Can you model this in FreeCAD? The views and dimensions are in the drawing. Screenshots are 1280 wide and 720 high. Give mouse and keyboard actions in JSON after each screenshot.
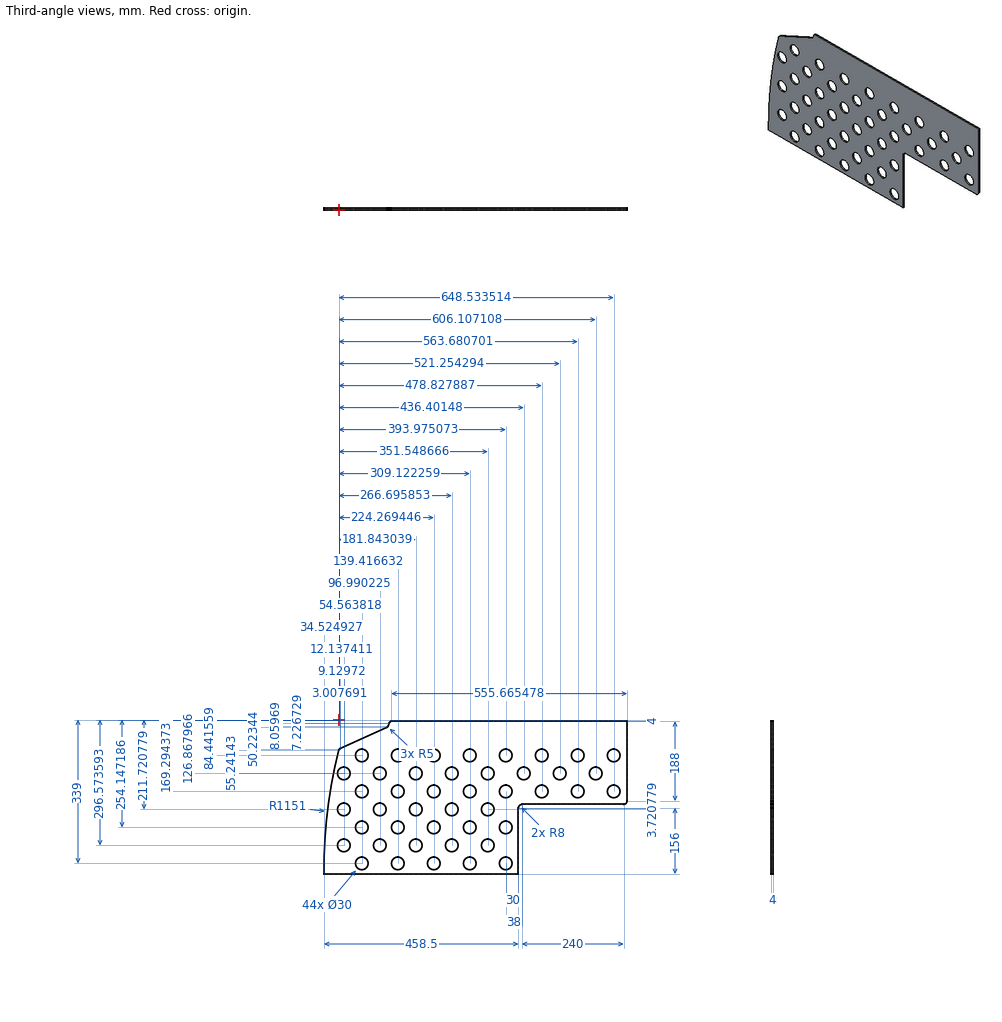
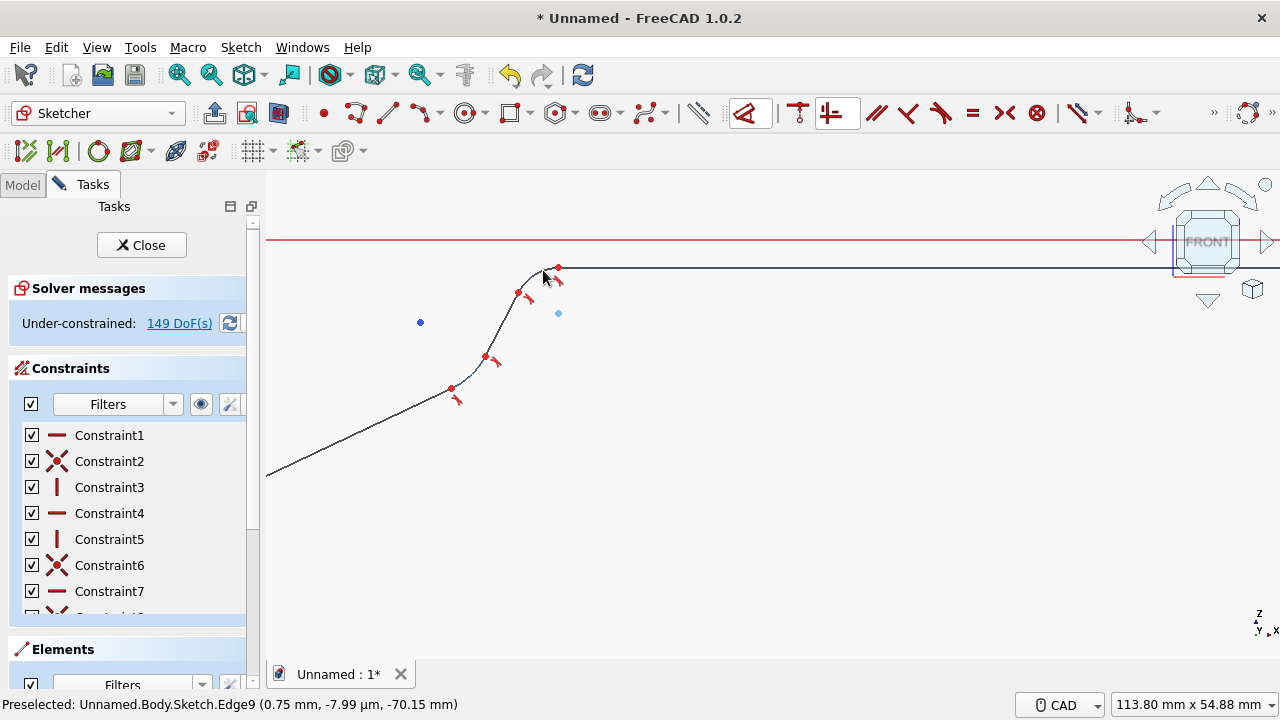
{"action": "left_click", "coordinate": [544, 270]}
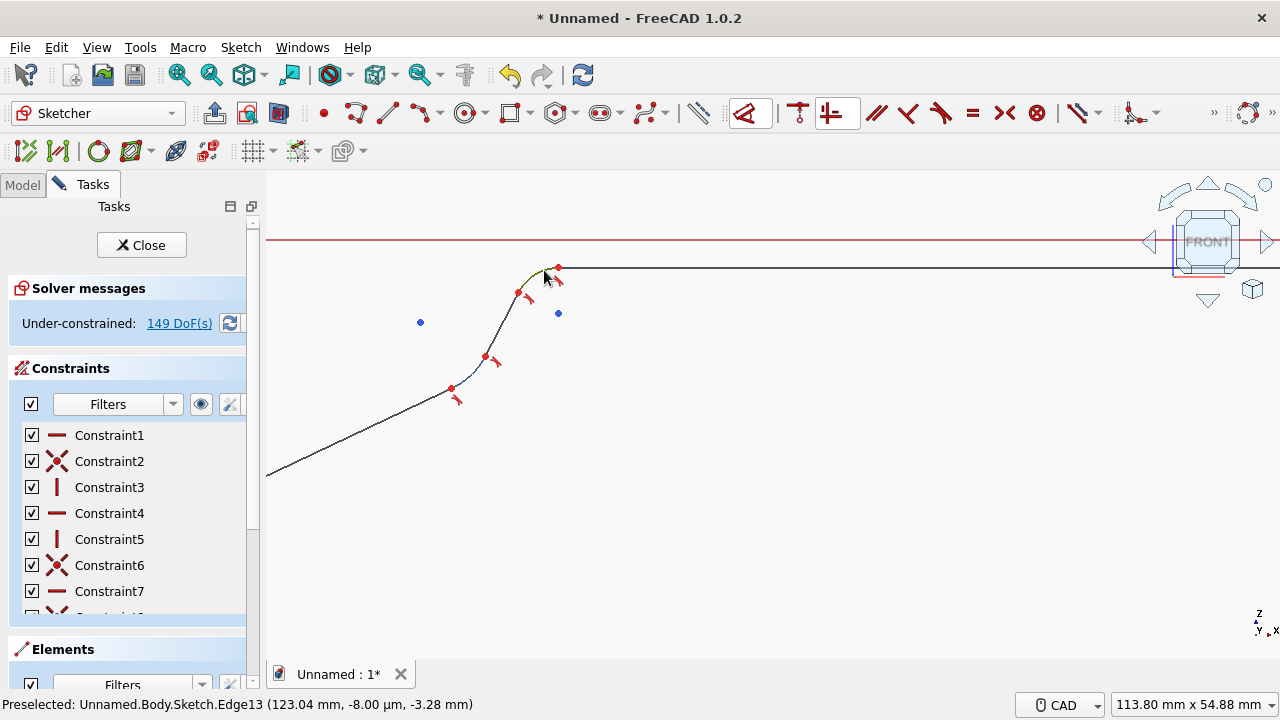
{"action": "left_click", "coordinate": [974, 114]}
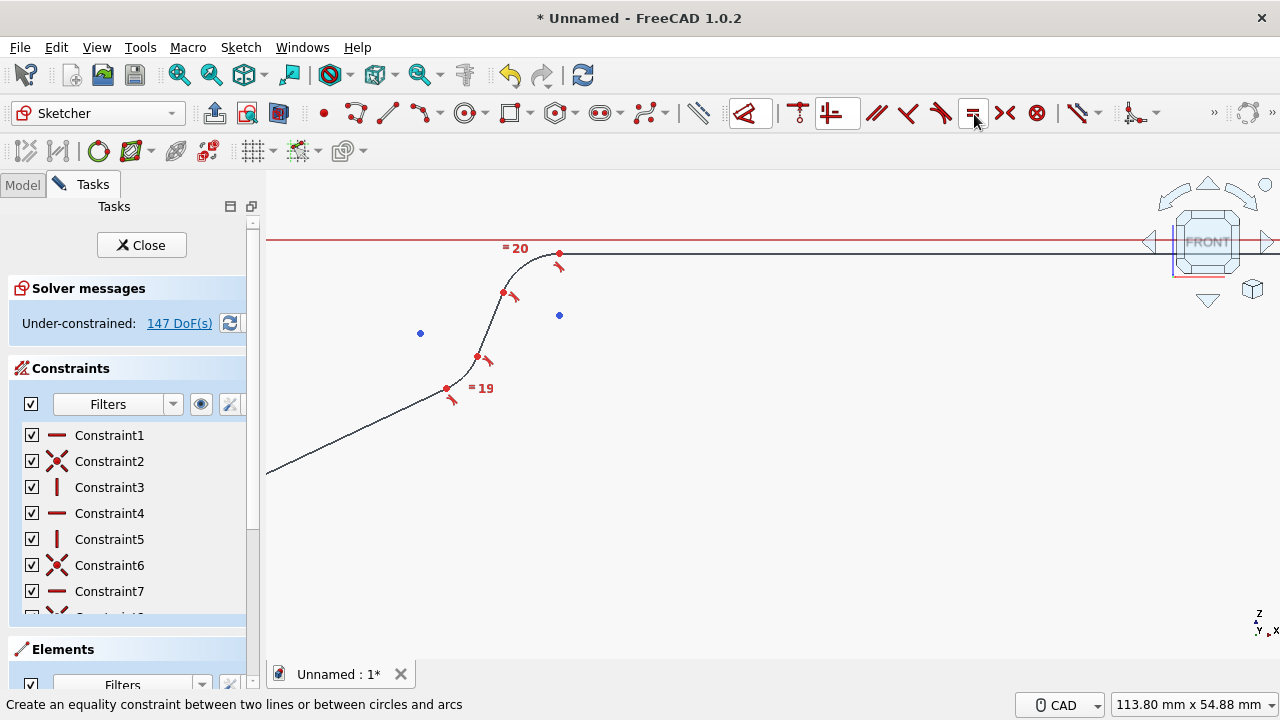
{"action": "scroll", "coordinate": [543, 270], "scroll_direction": "down", "scroll_amount": 12}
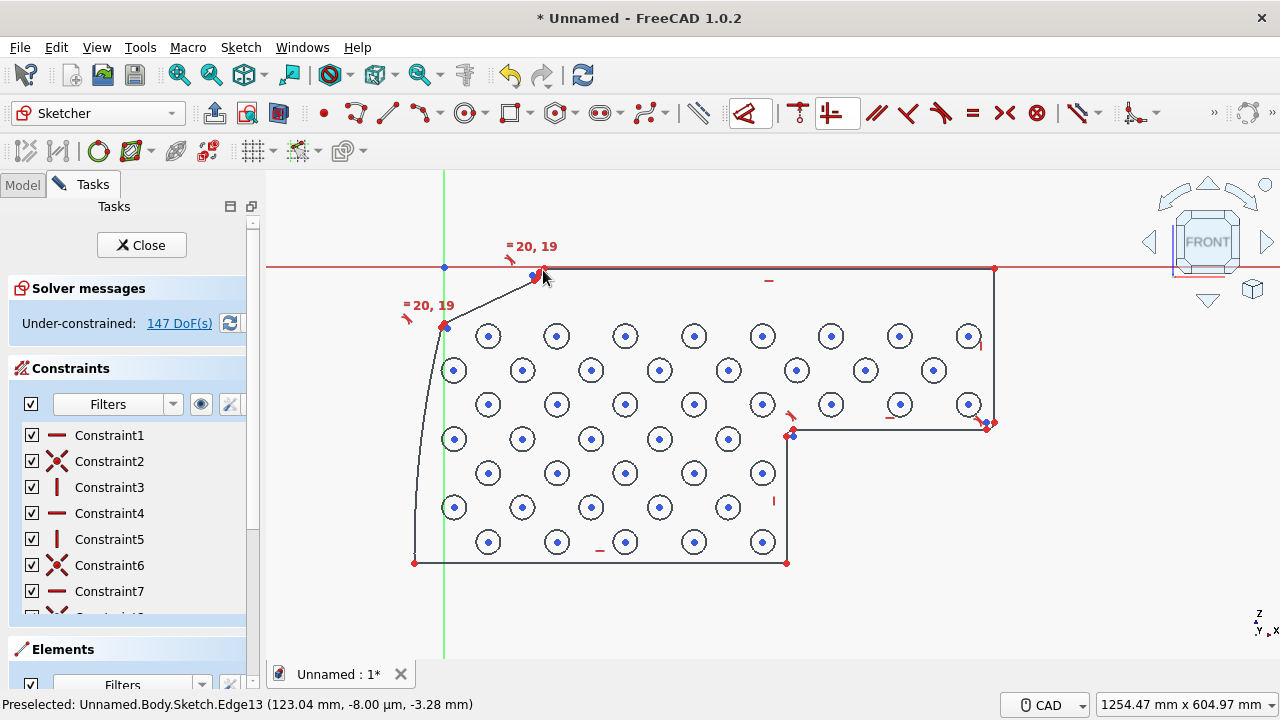
{"action": "scroll", "coordinate": [790, 431], "scroll_direction": "up", "scroll_amount": 8}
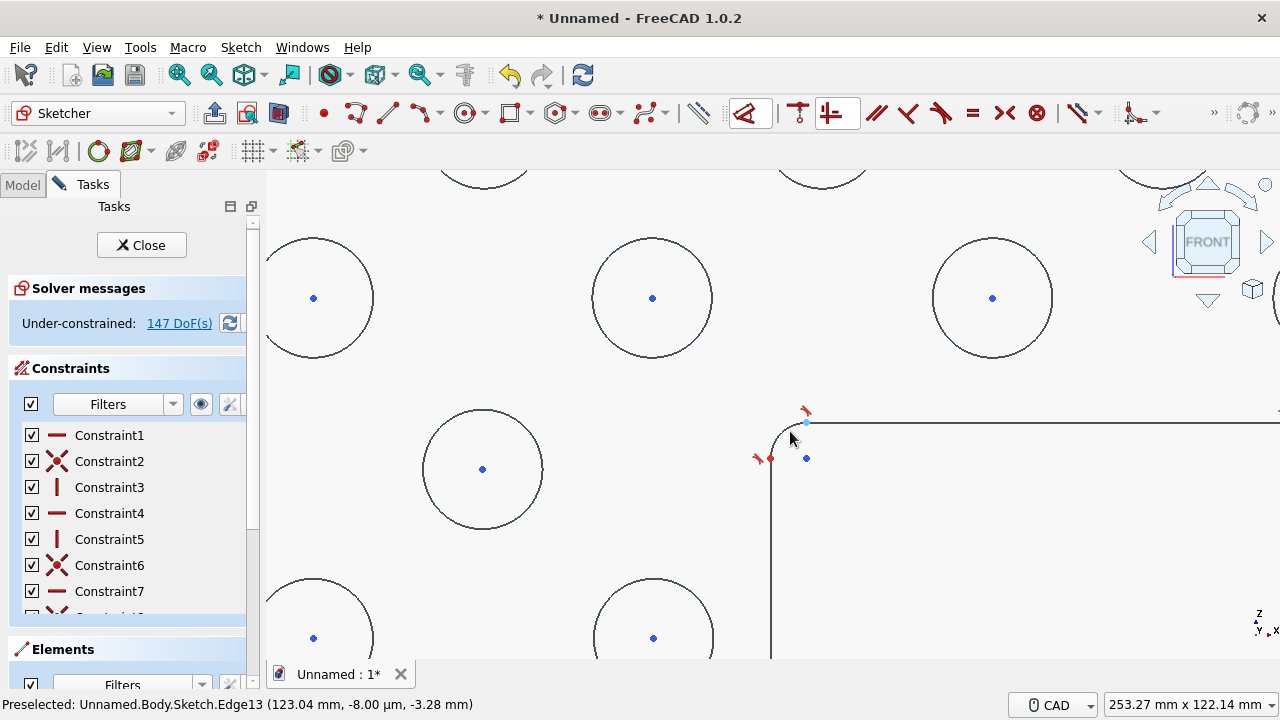
{"action": "left_click", "coordinate": [790, 427]}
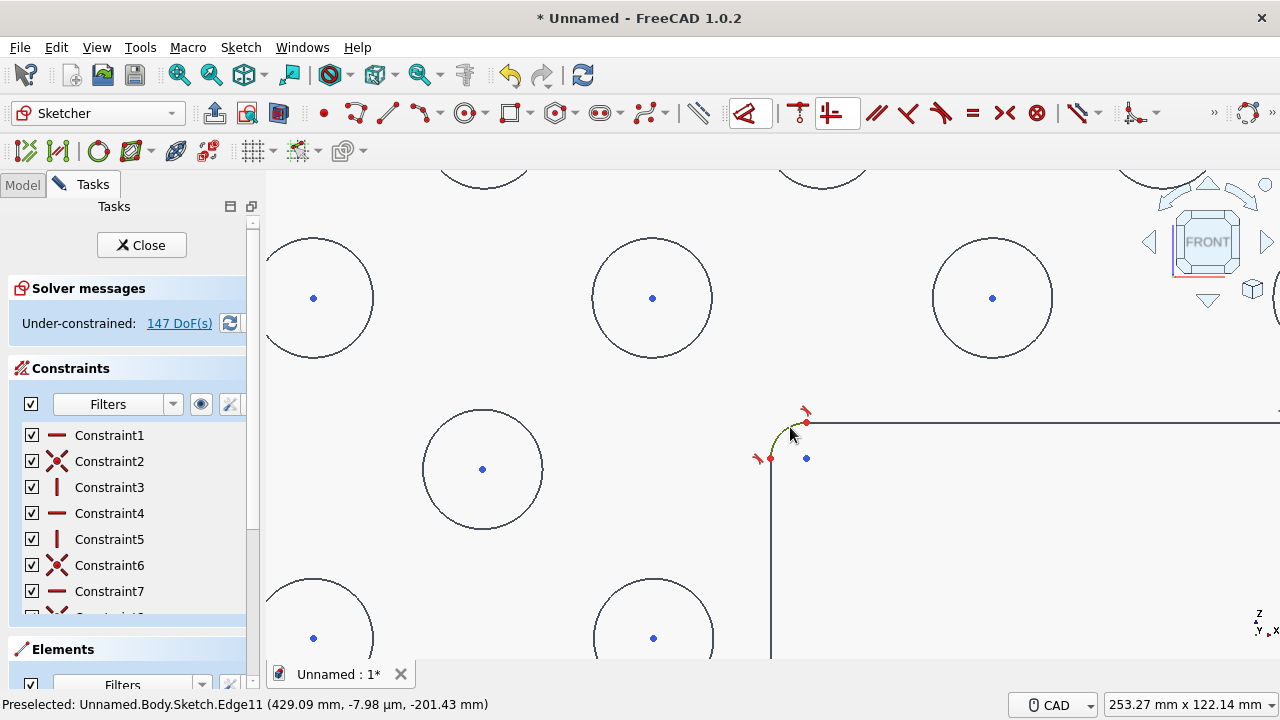
{"action": "scroll", "coordinate": [790, 431], "scroll_direction": "down", "scroll_amount": 8}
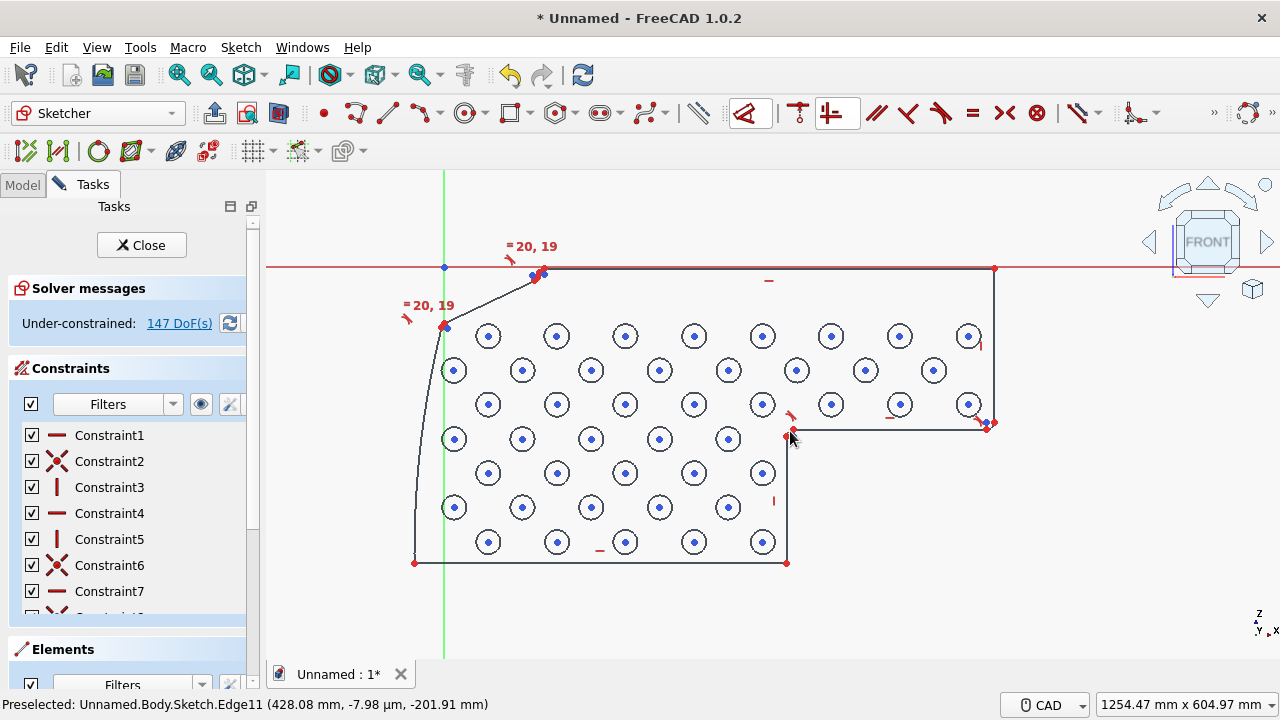
{"action": "scroll", "coordinate": [990, 429], "scroll_direction": "up", "scroll_amount": 7}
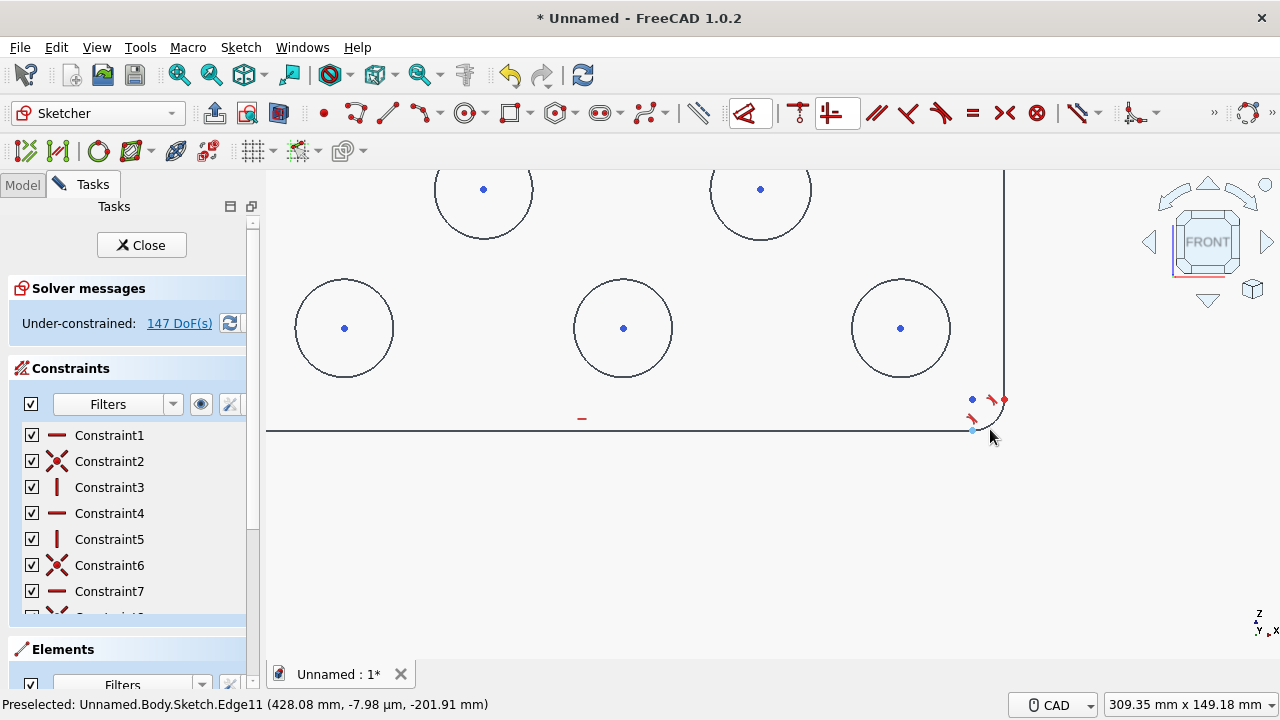
{"action": "left_click", "coordinate": [987, 427]}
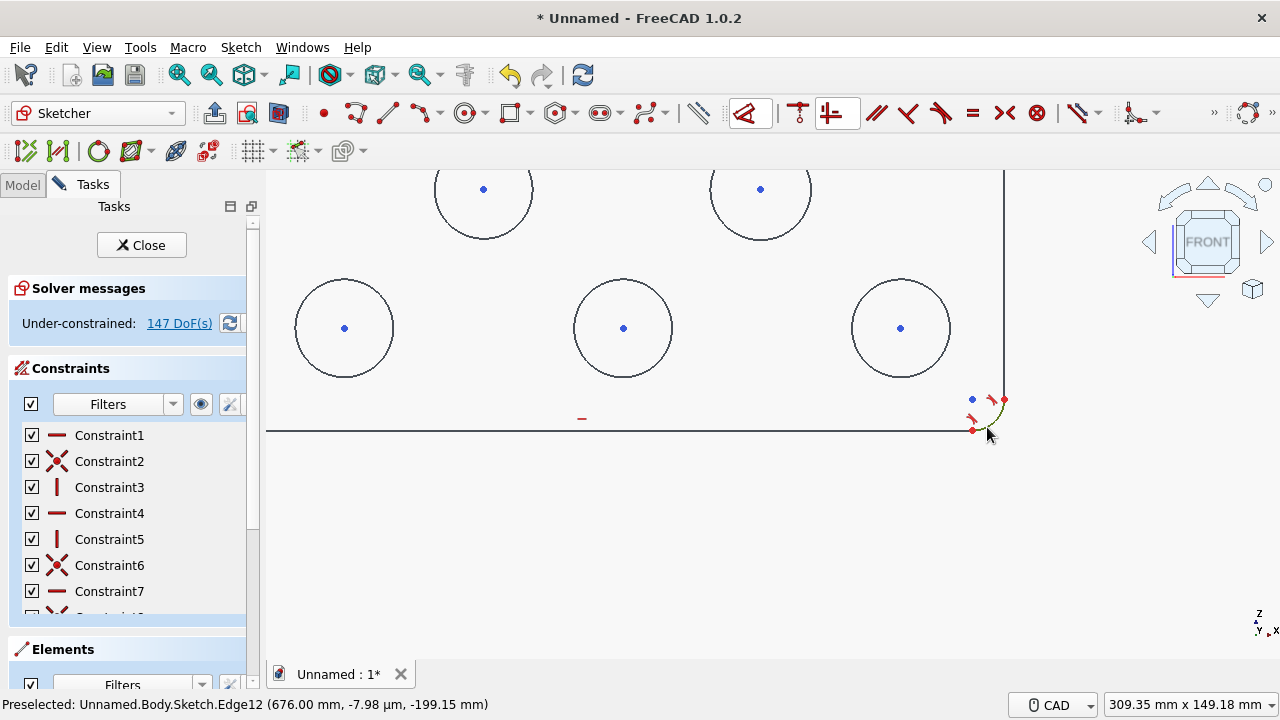
{"action": "key", "text": "e"}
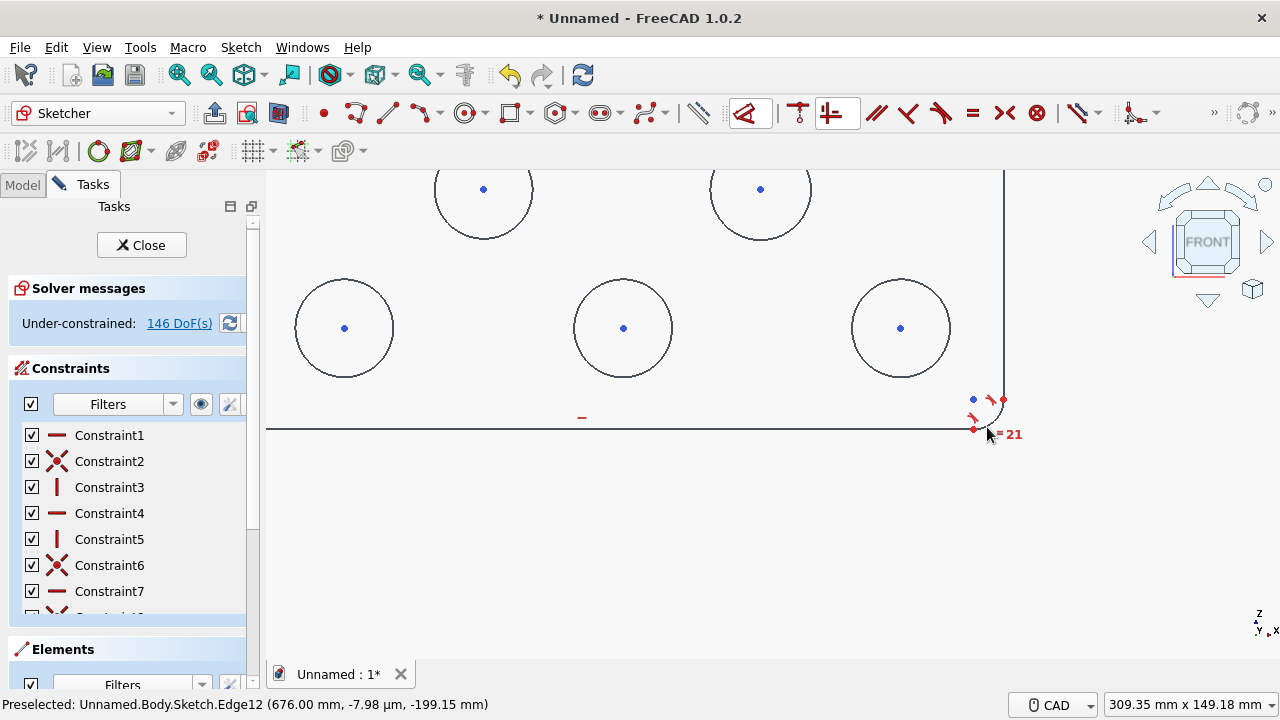
{"action": "scroll", "coordinate": [990, 429], "scroll_direction": "down", "scroll_amount": 7}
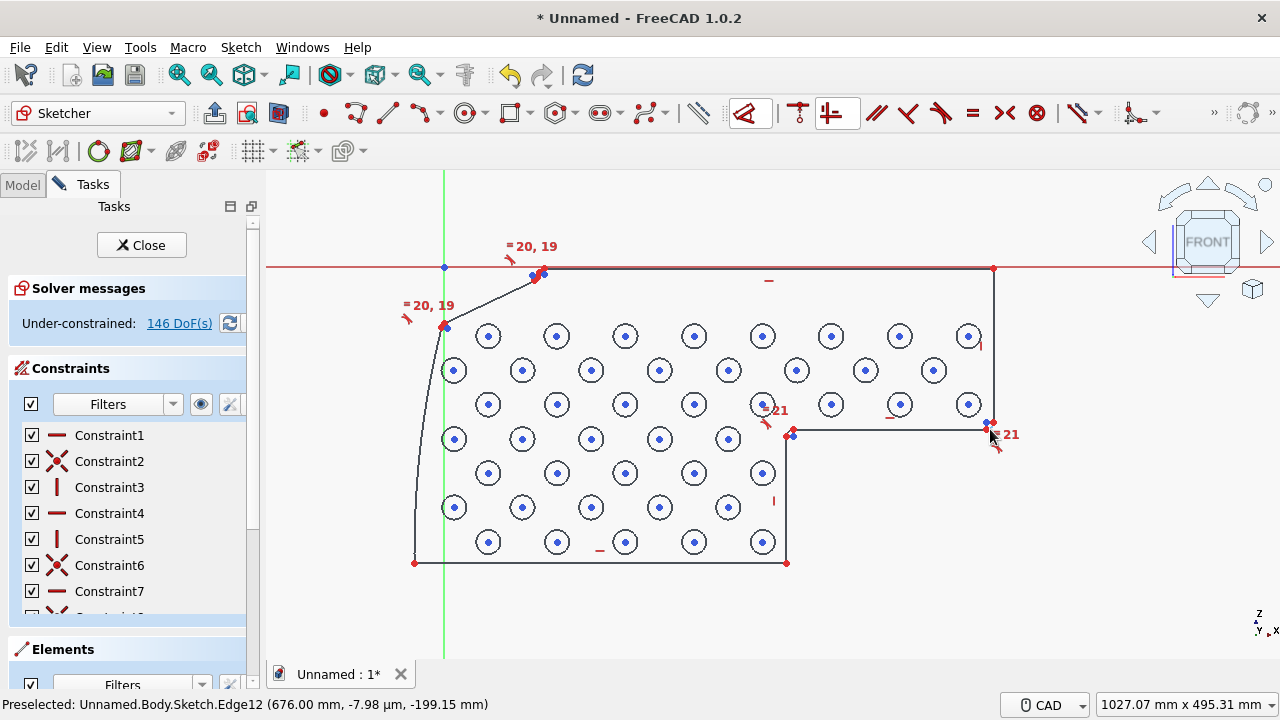
{"action": "left_click", "coordinate": [497, 534]}